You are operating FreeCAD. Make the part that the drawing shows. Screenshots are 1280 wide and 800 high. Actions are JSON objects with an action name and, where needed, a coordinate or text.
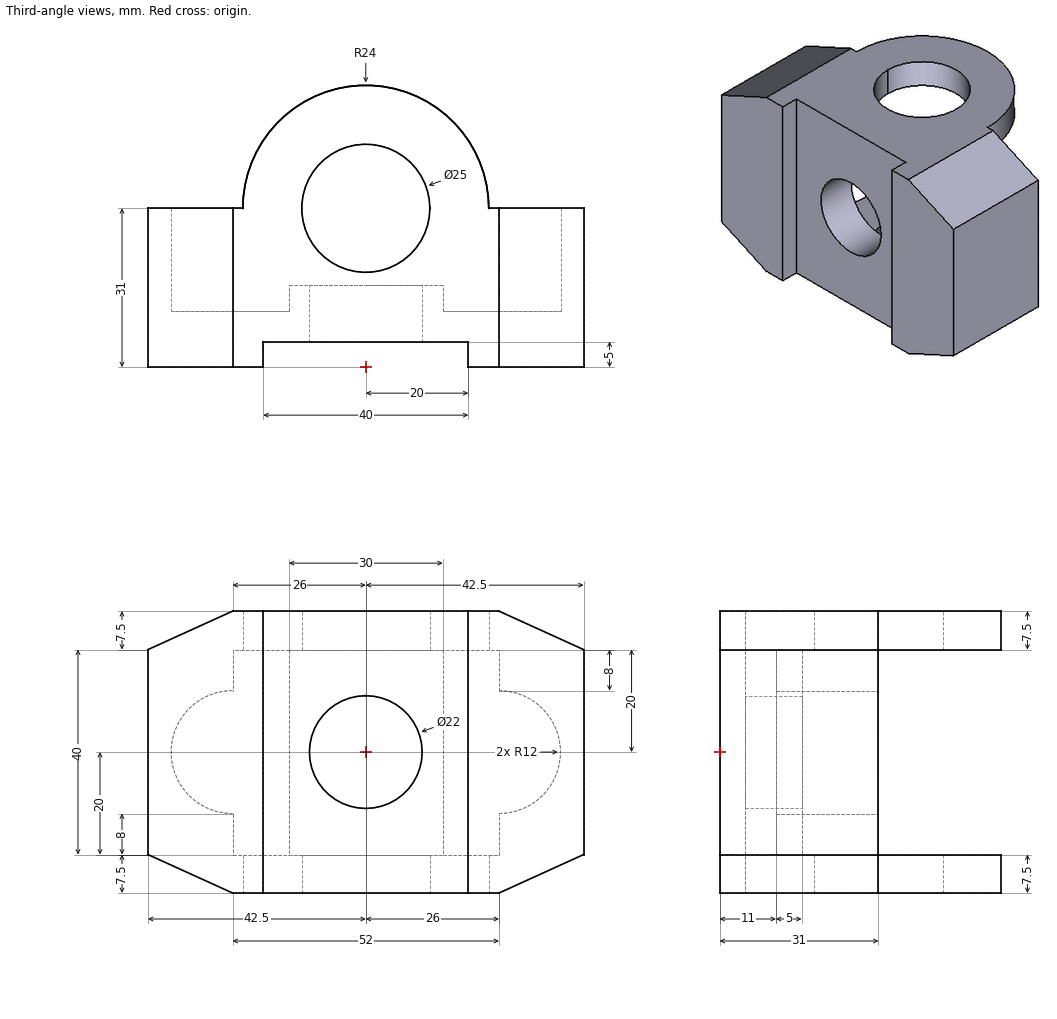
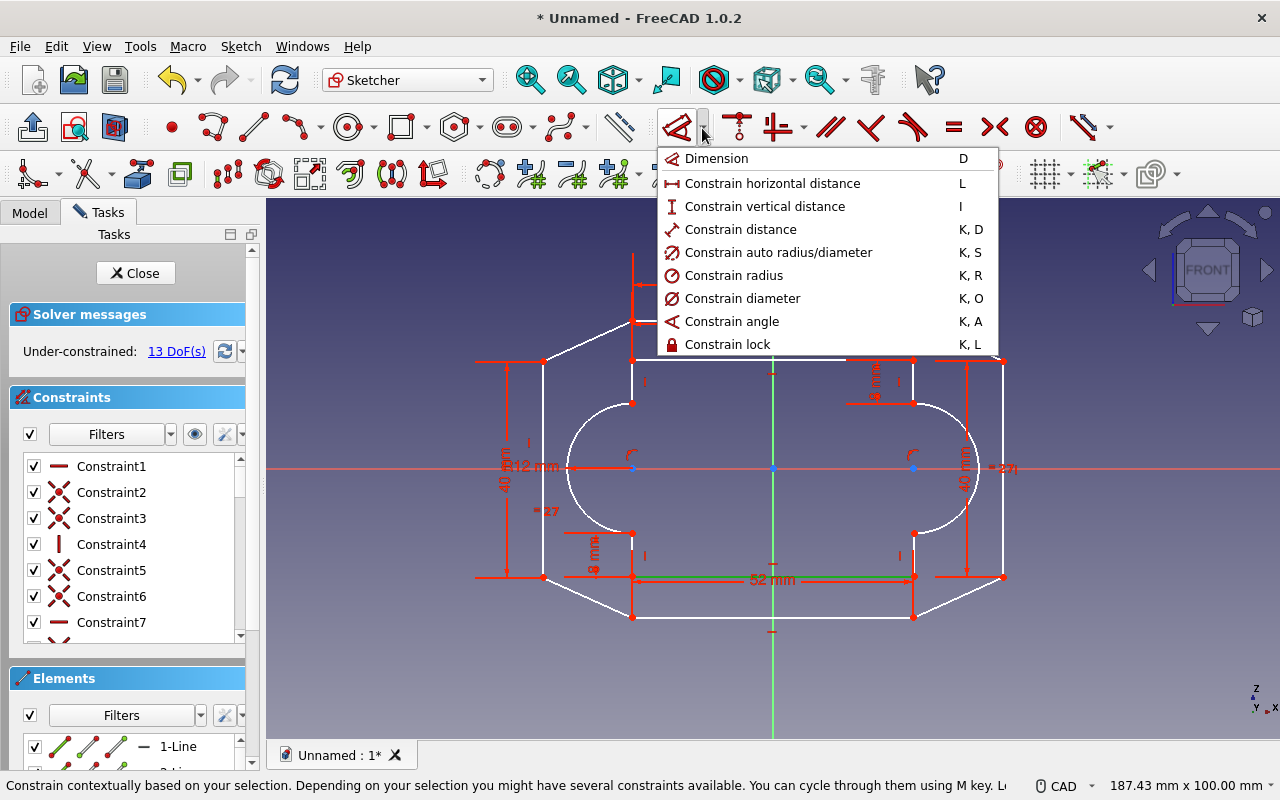
{"action": "left_click", "coordinate": [828, 184]}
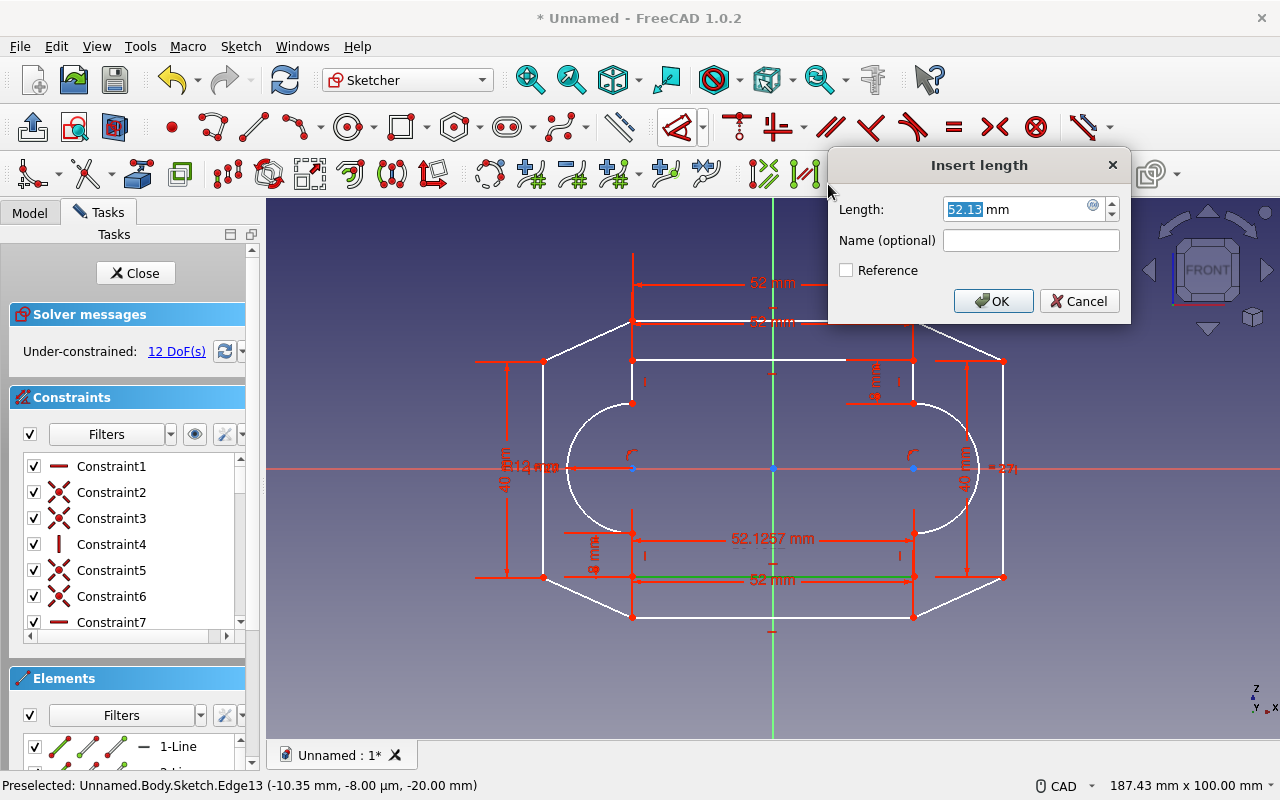
{"action": "type", "text": "52"}
{"action": "key", "text": "Return"}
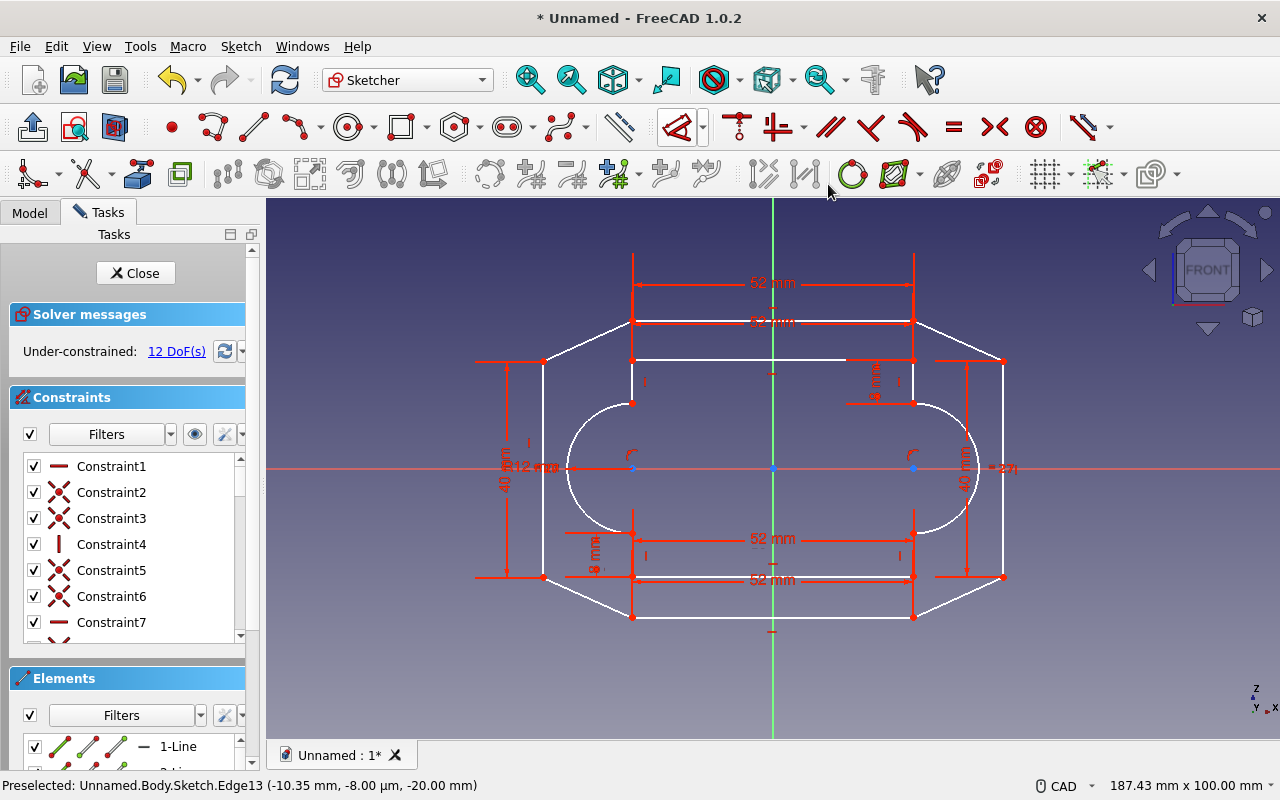
{"action": "left_click", "coordinate": [913, 618]}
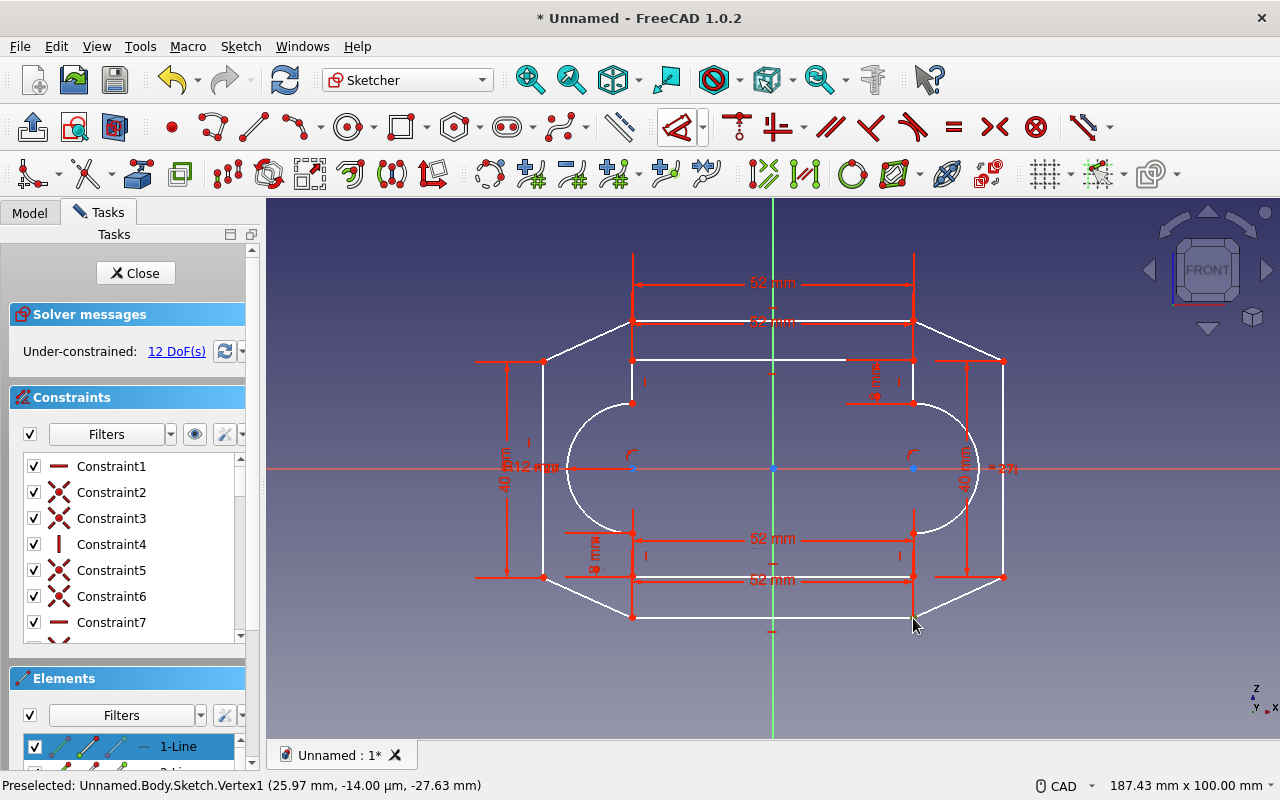
{"action": "key", "text": "l"}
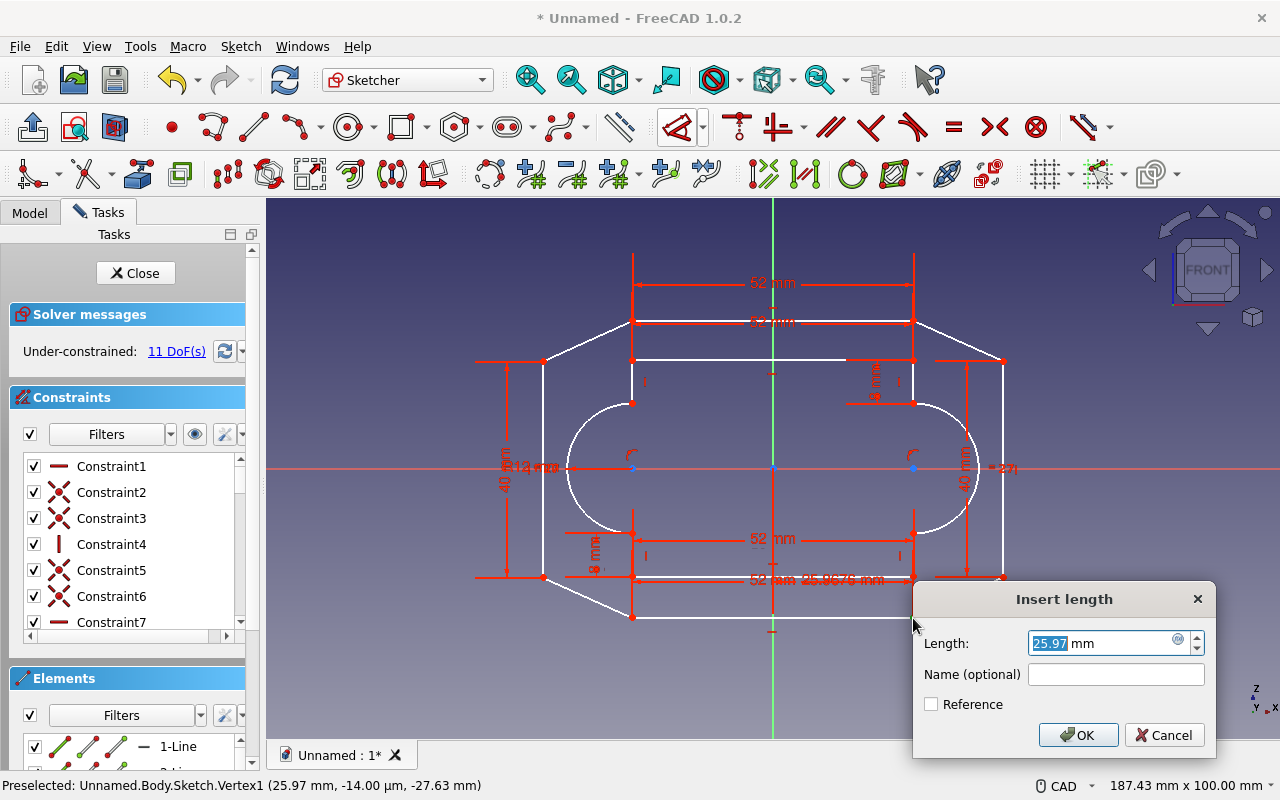
{"action": "type", "text": "26"}
{"action": "key", "text": "Return"}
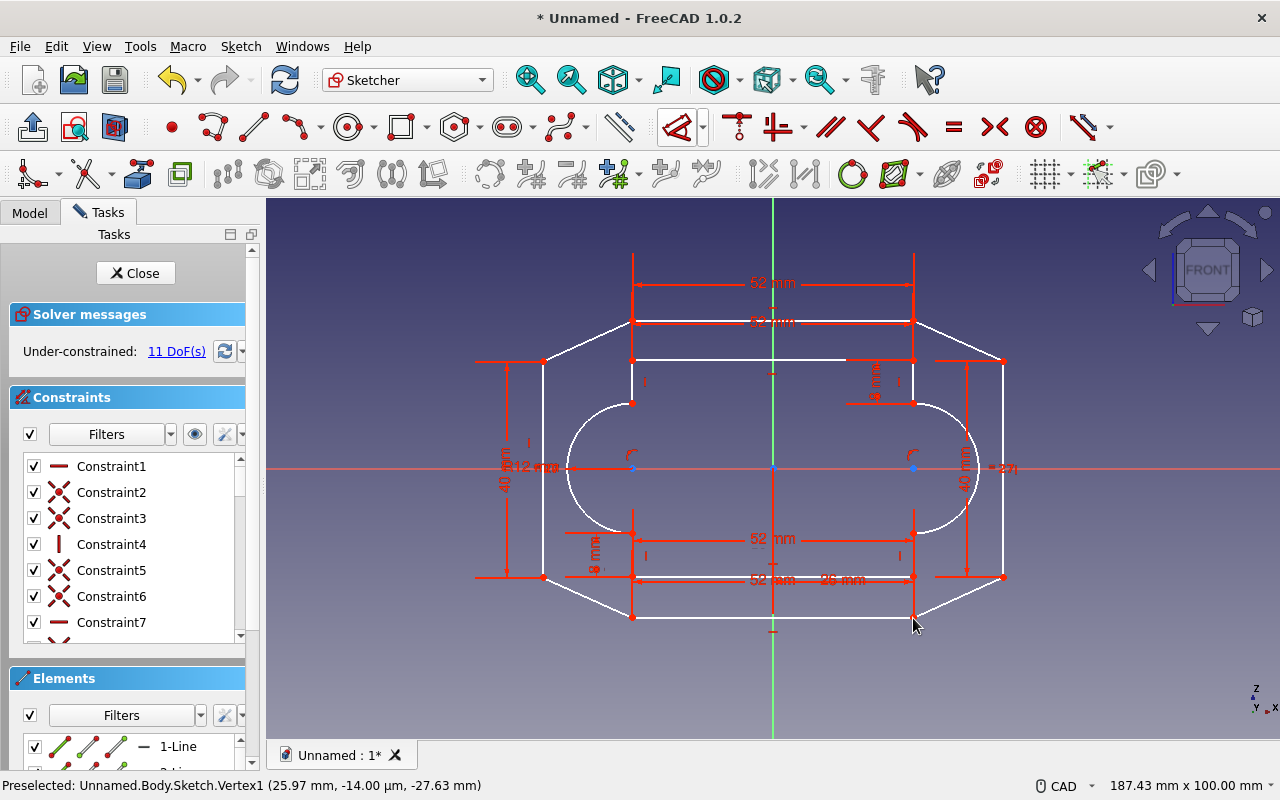
{"action": "left_click", "coordinate": [543, 578]}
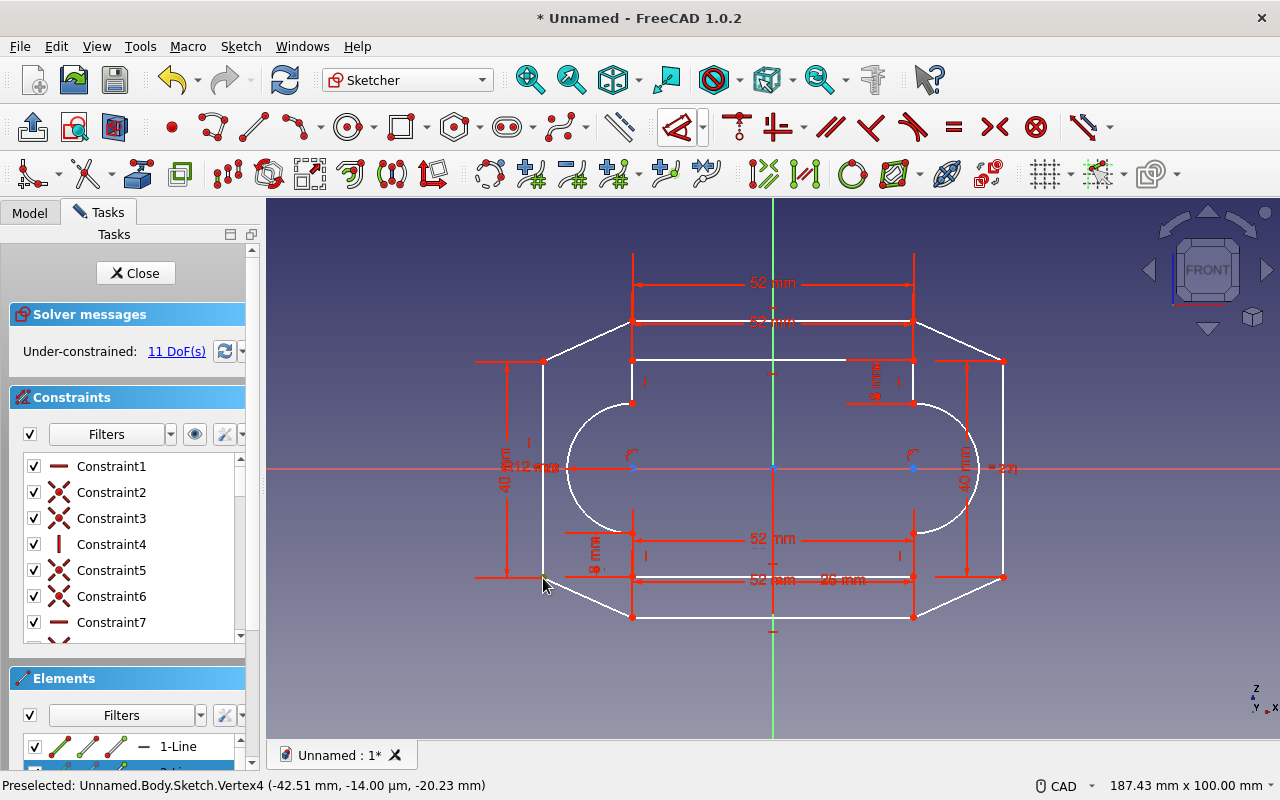
{"action": "key", "text": "i"}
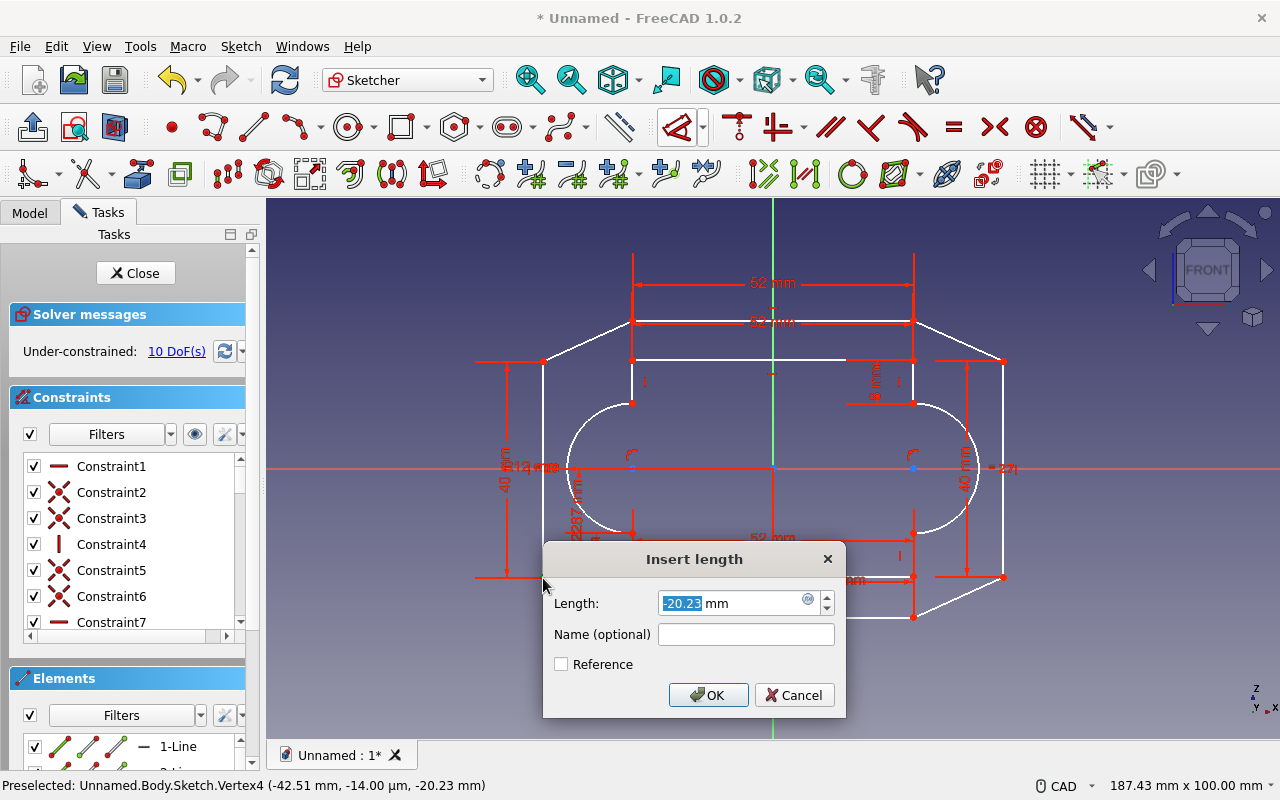
{"action": "type", "text": "-20"}
{"action": "key", "text": "Return"}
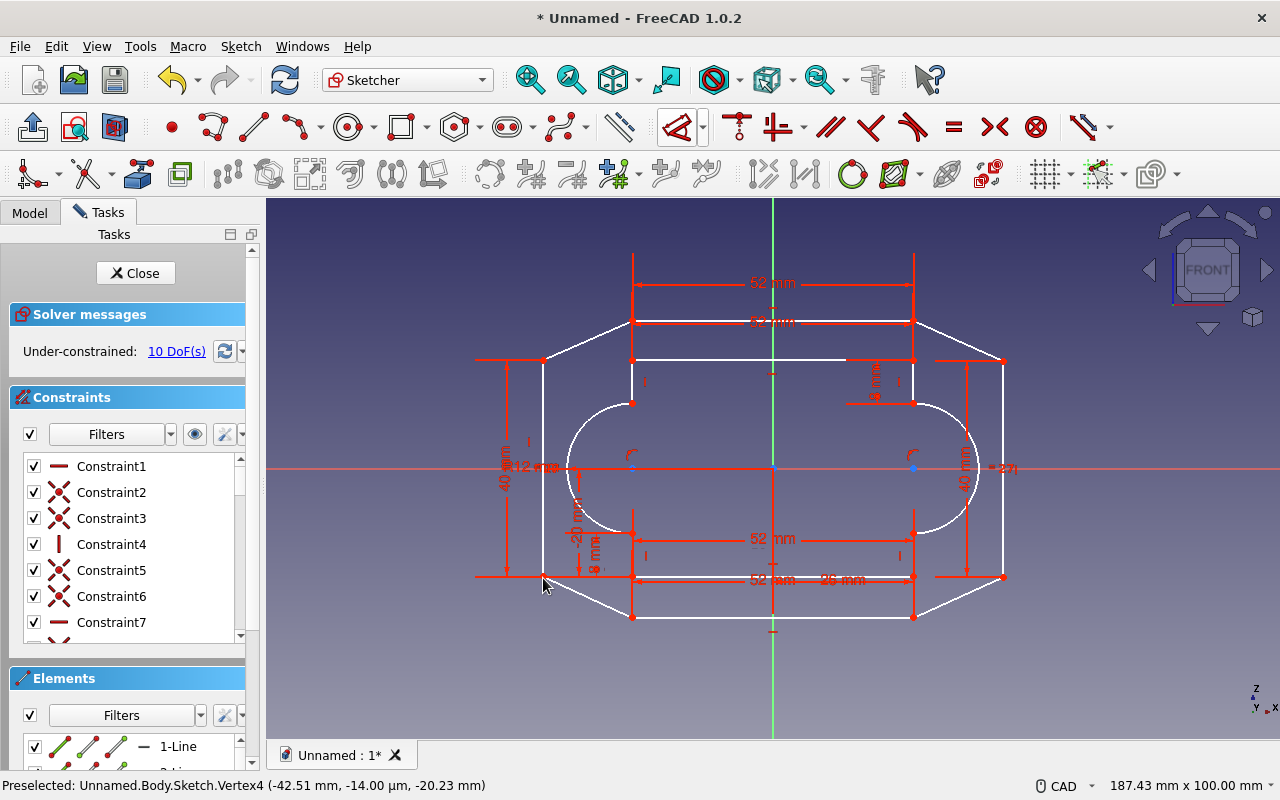
{"action": "left_click", "coordinate": [633, 321]}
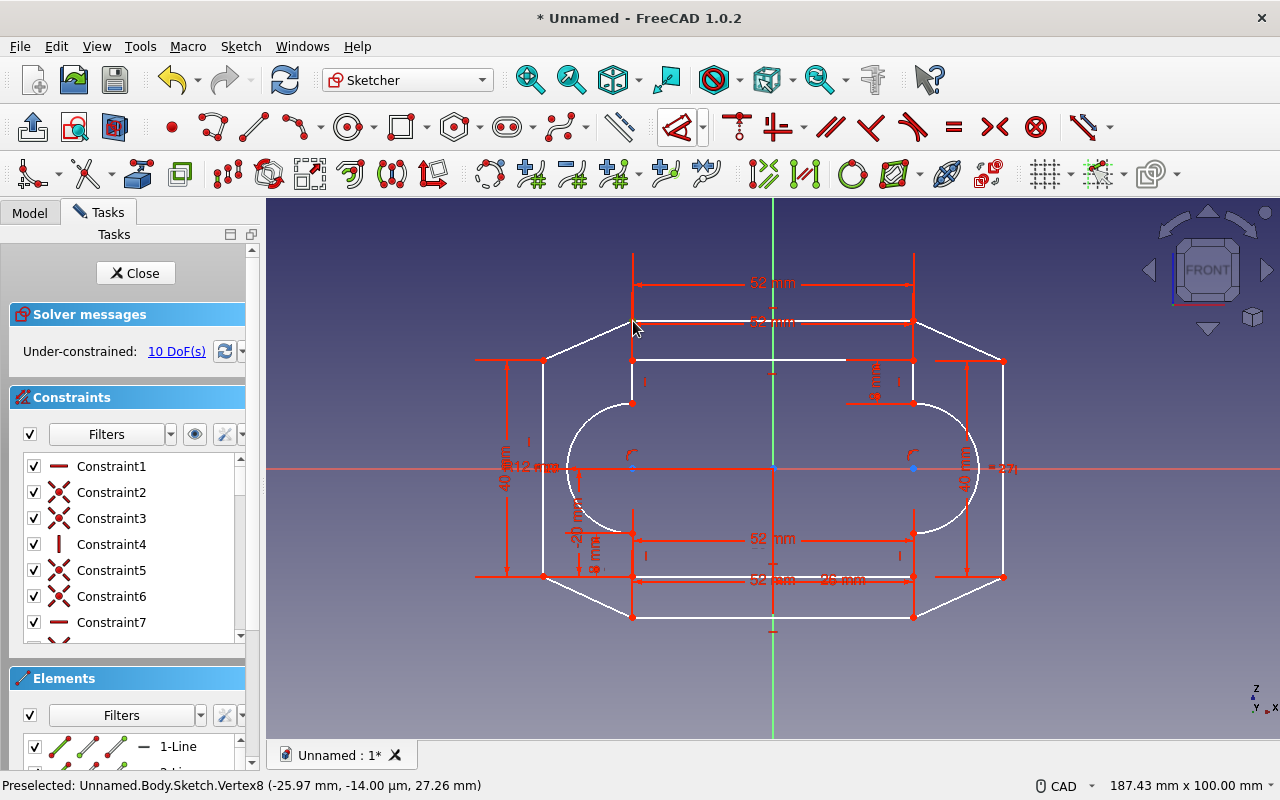
{"action": "left_click", "coordinate": [702, 128]}